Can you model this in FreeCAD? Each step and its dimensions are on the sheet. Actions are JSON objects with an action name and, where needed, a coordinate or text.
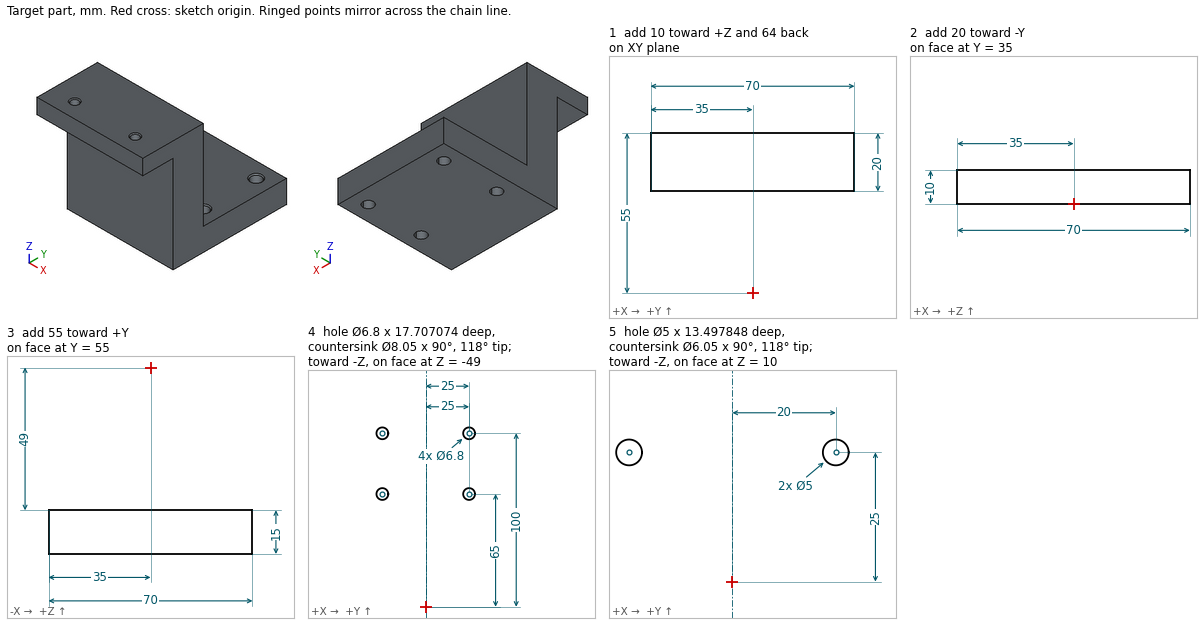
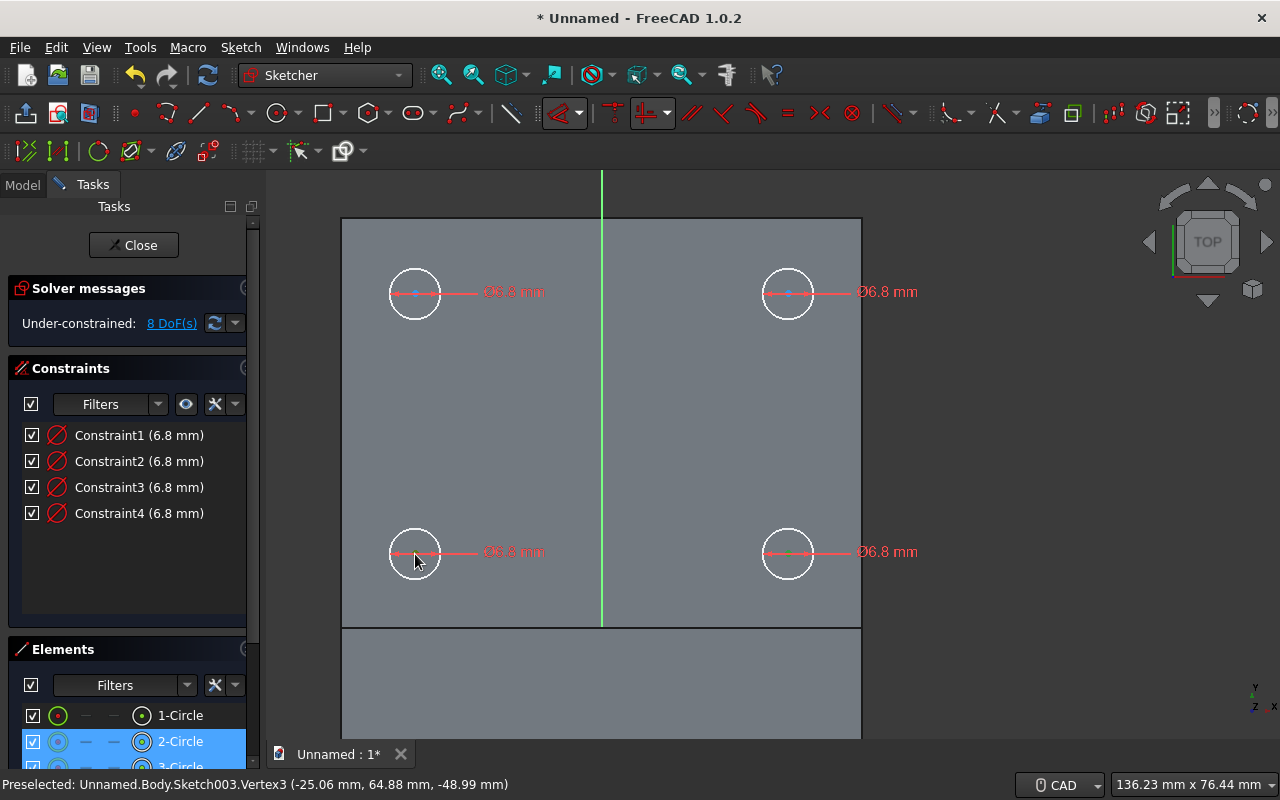
{"action": "left_click", "coordinate": [602, 674]}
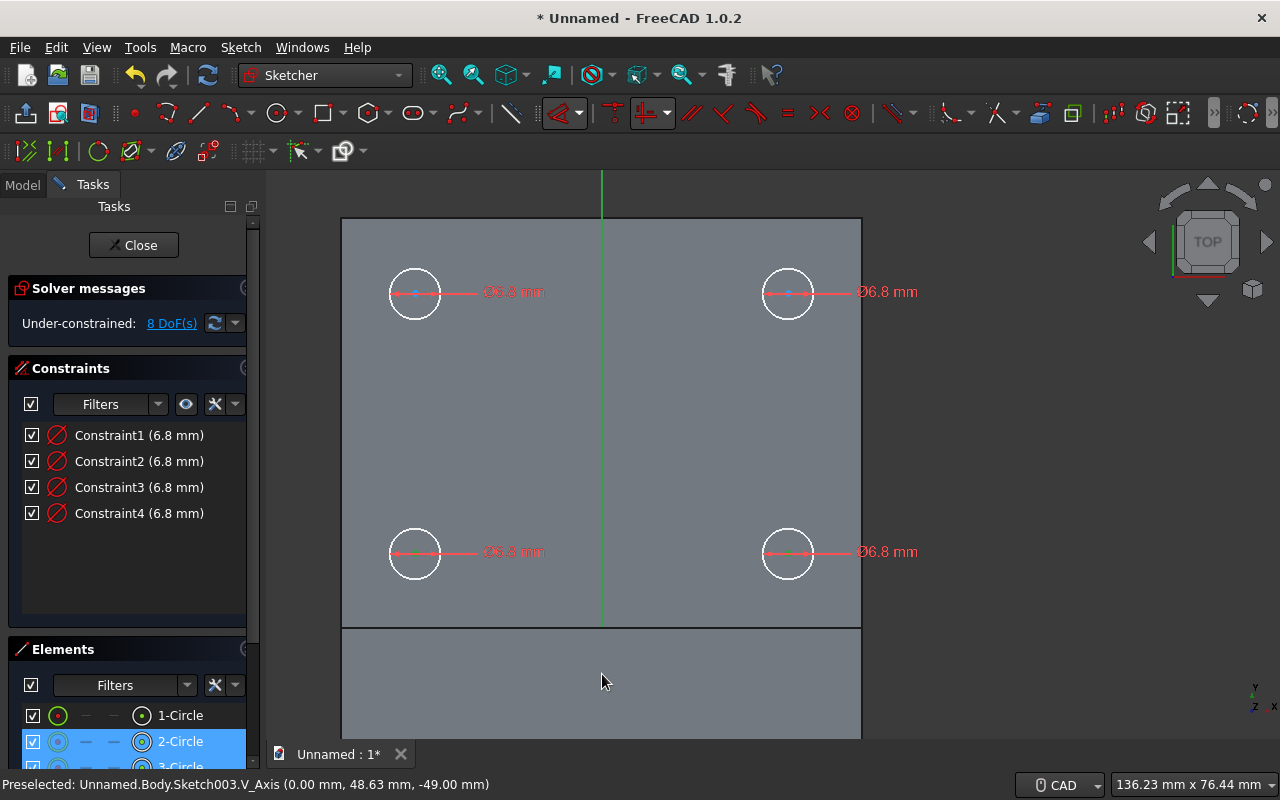
{"action": "left_click", "coordinate": [820, 114]}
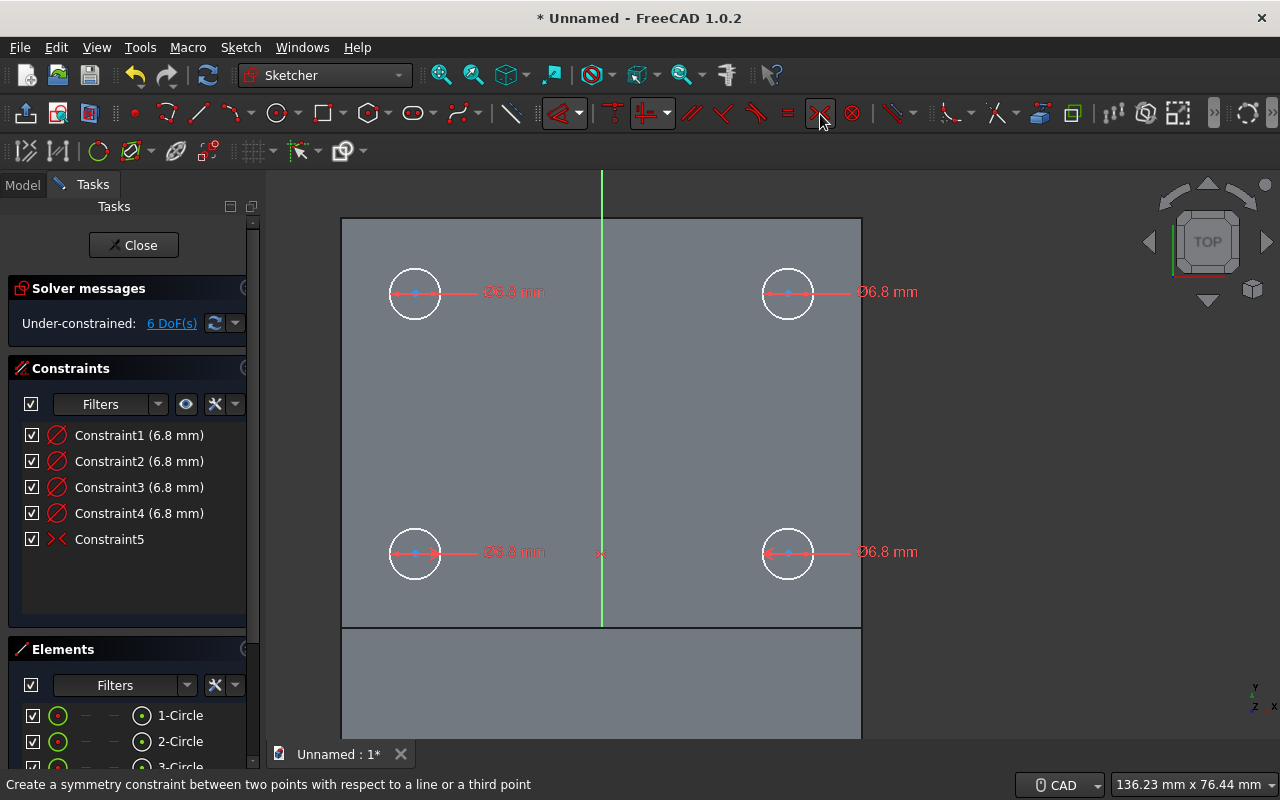
{"action": "left_click", "coordinate": [788, 294]}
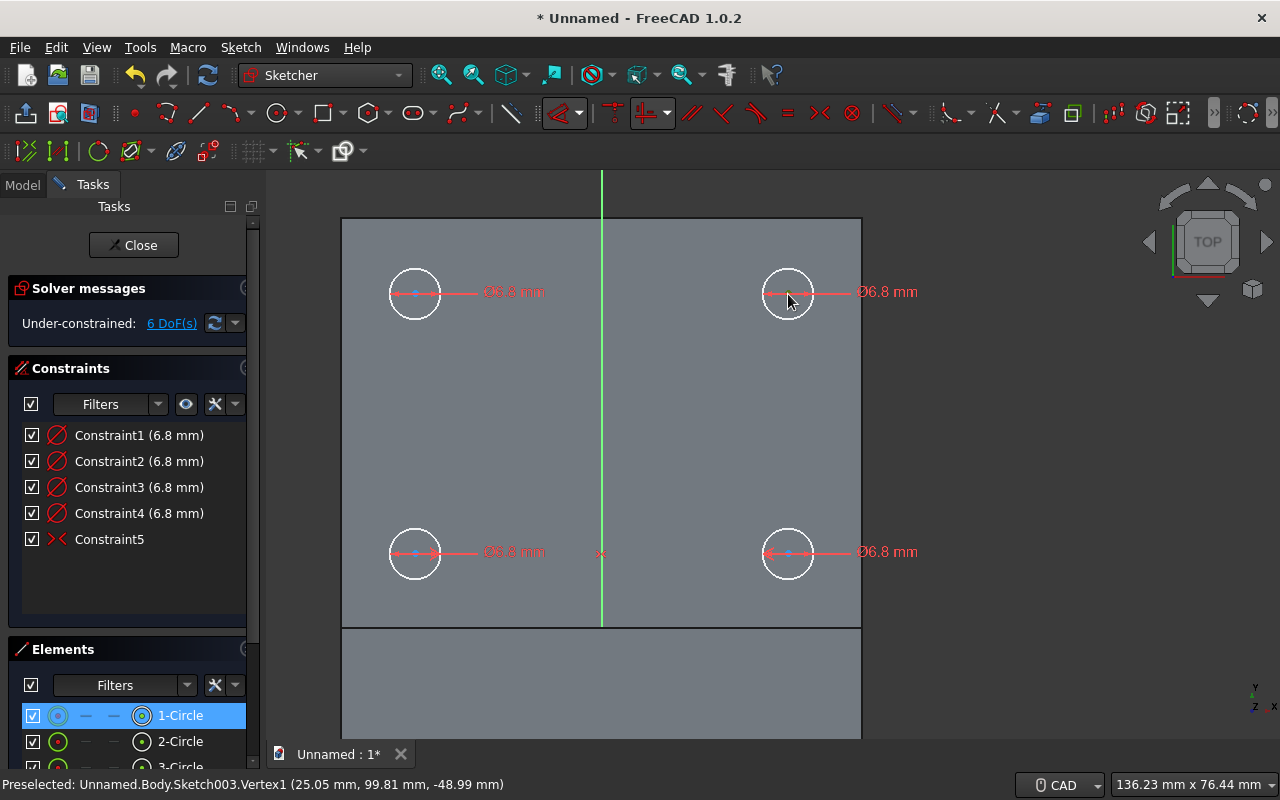
{"action": "left_click", "coordinate": [415, 294]}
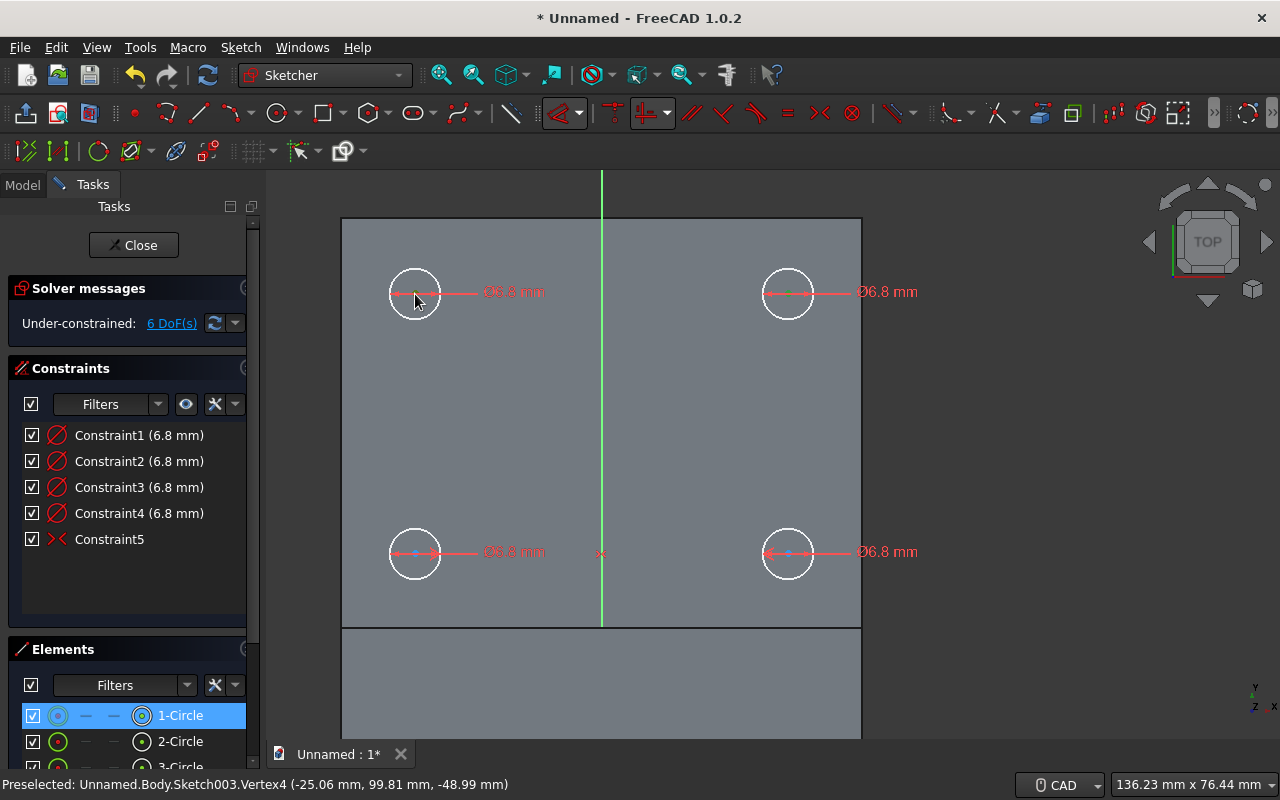
{"action": "left_click", "coordinate": [602, 674]}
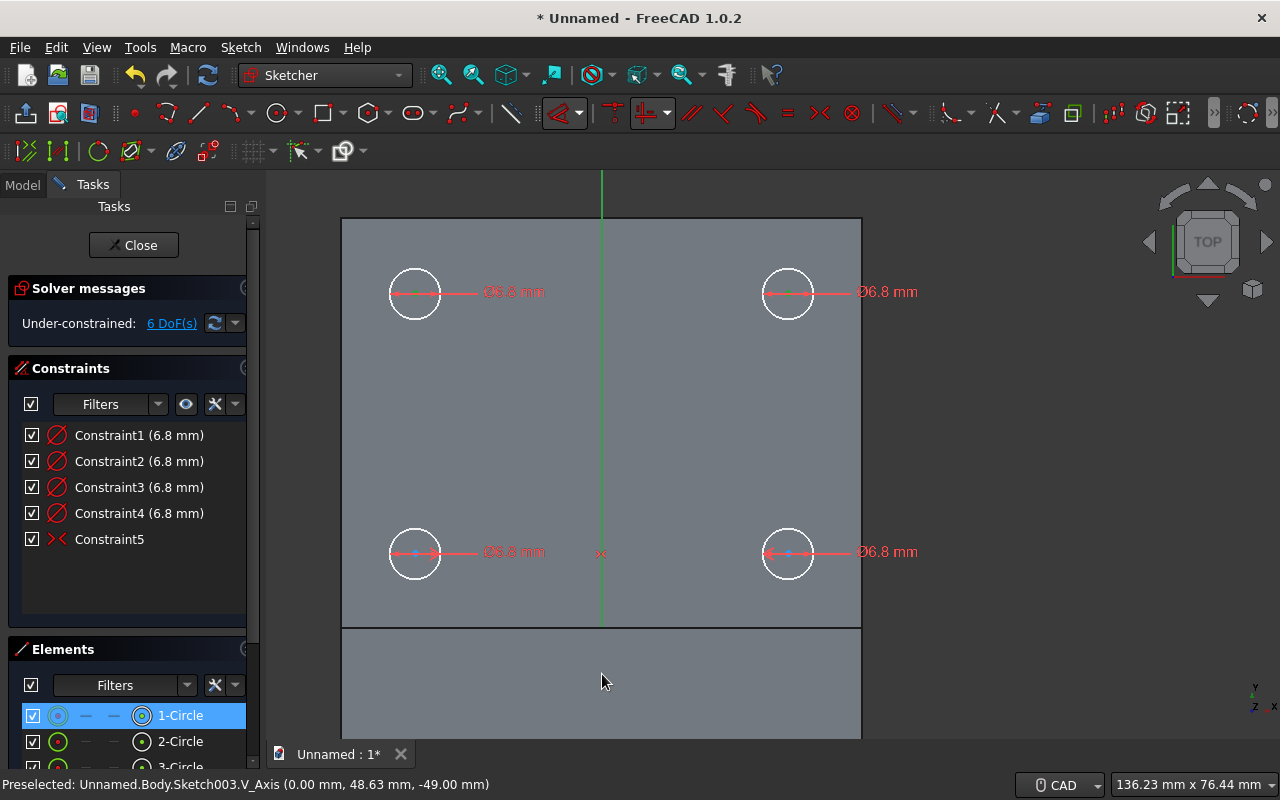
{"action": "key", "text": "s"}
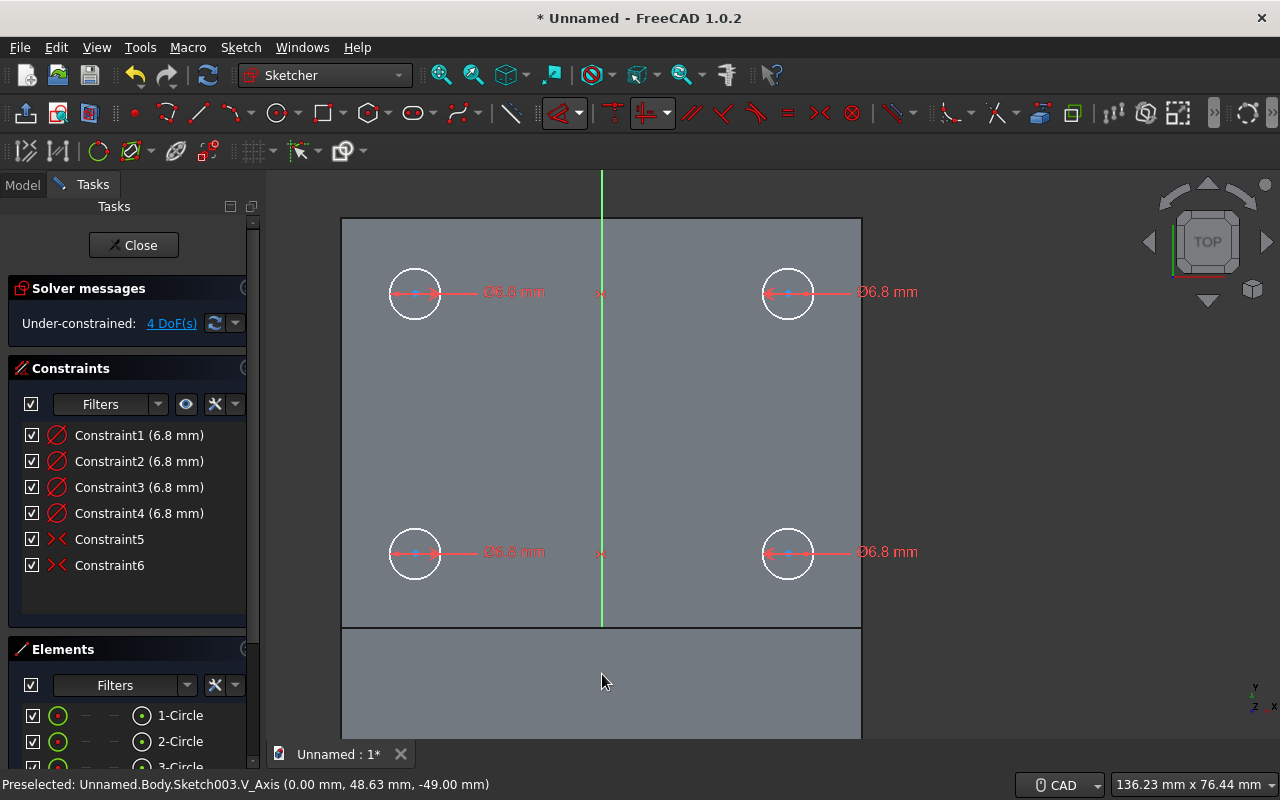
{"action": "left_click", "coordinate": [788, 294]}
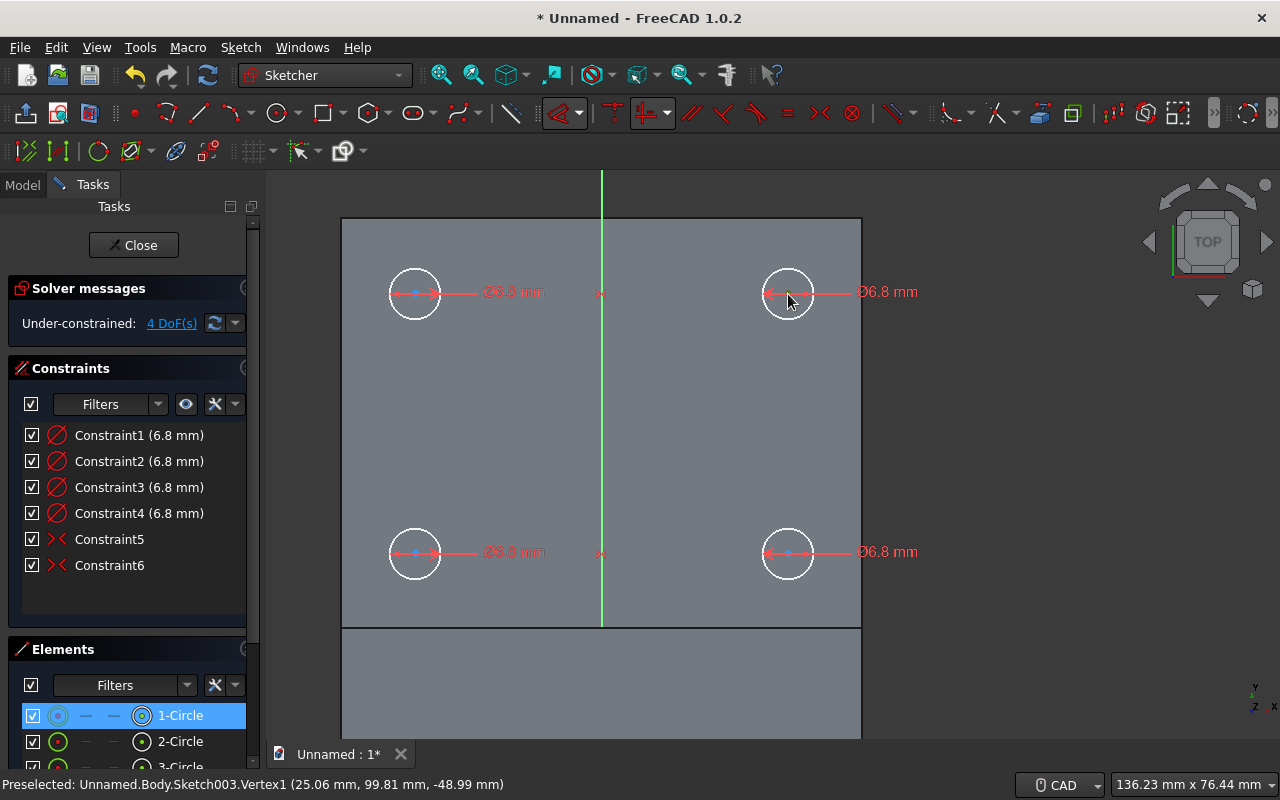
{"action": "left_click", "coordinate": [582, 114]}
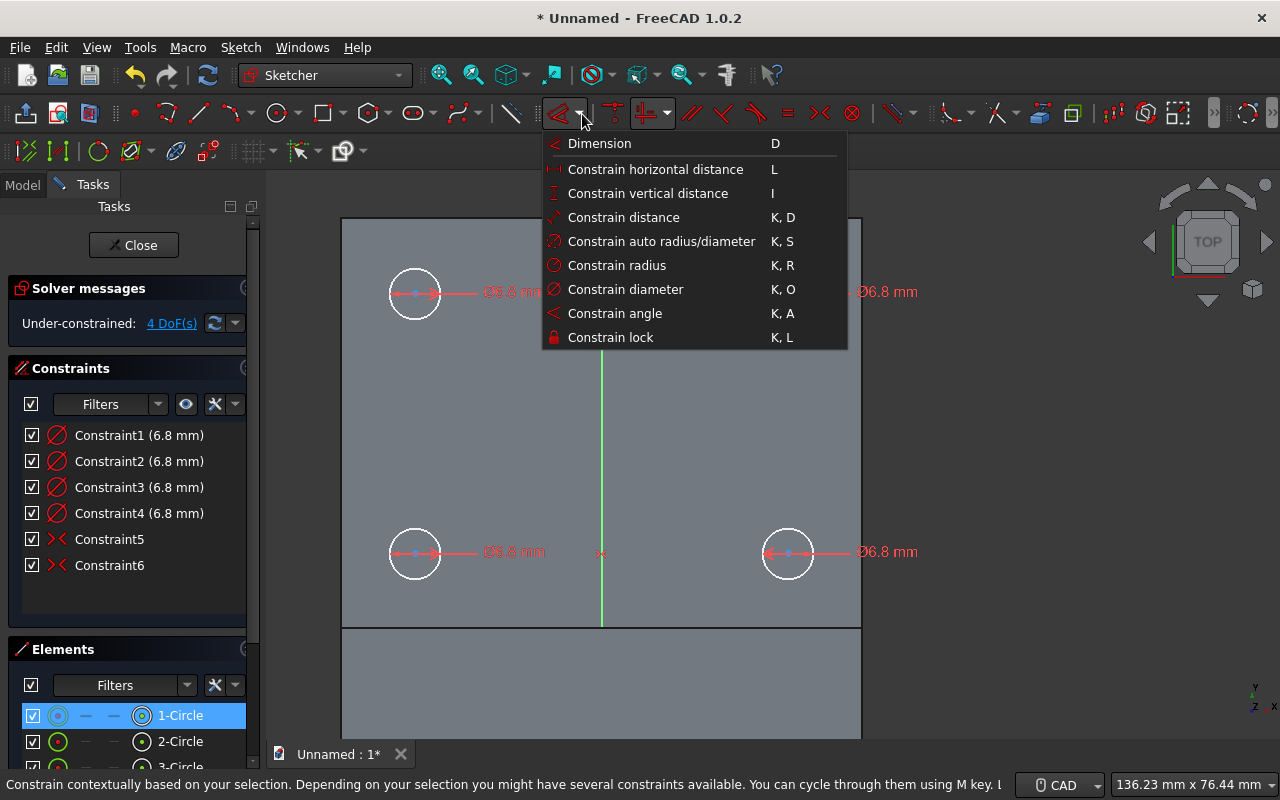
{"action": "left_click", "coordinate": [695, 169]}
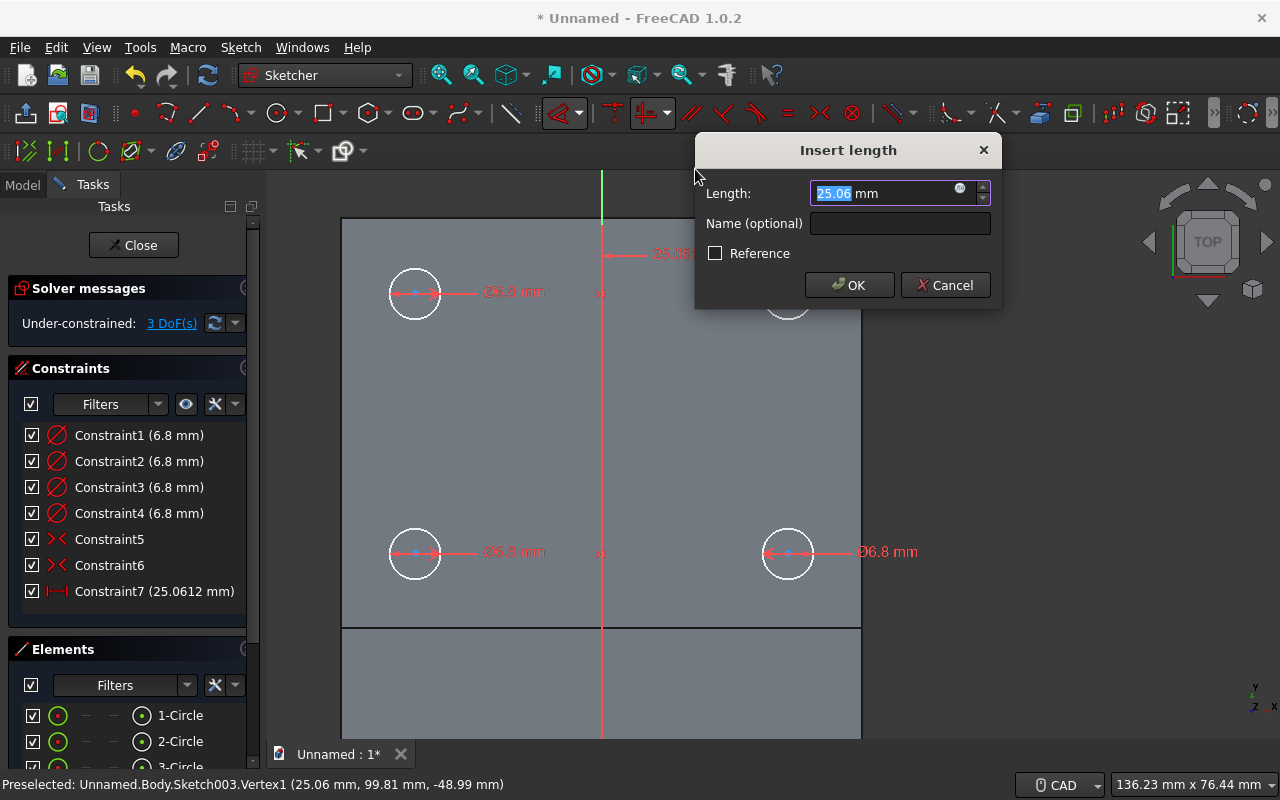
{"action": "type", "text": "25"}
{"action": "key", "text": "Return"}